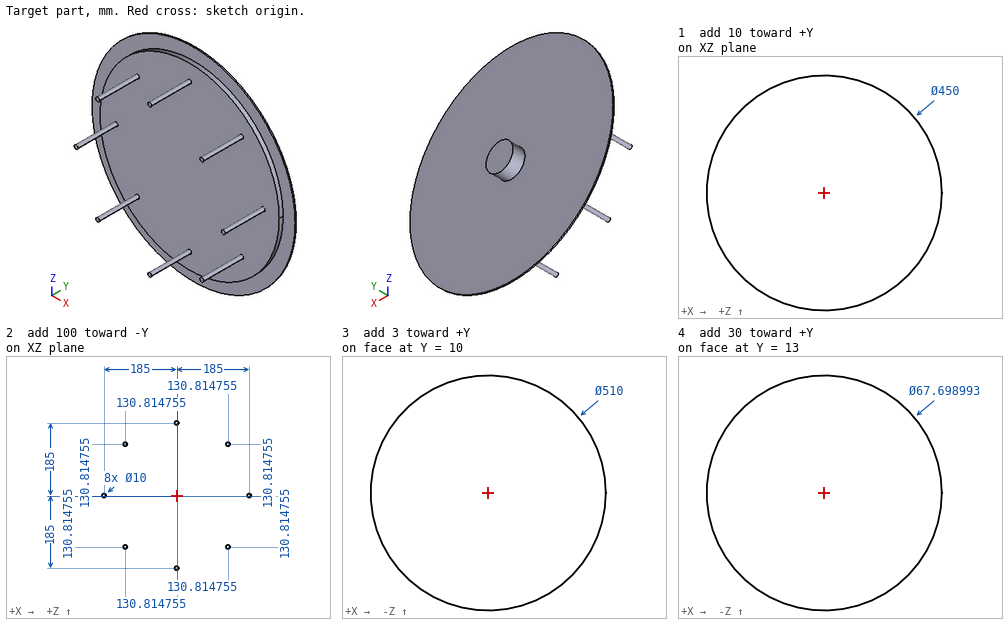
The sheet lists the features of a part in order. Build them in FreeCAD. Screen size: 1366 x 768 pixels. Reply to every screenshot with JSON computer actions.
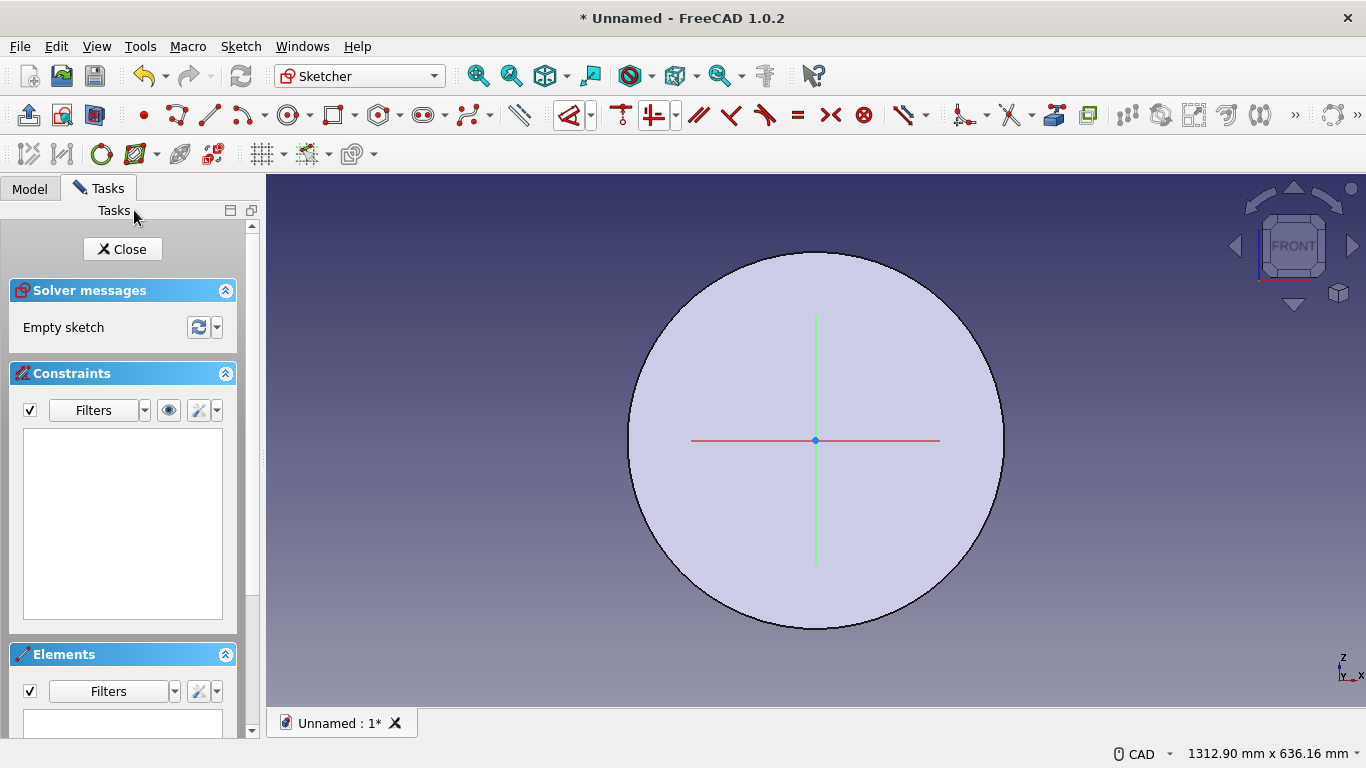
{"action": "left_click", "coordinate": [288, 116]}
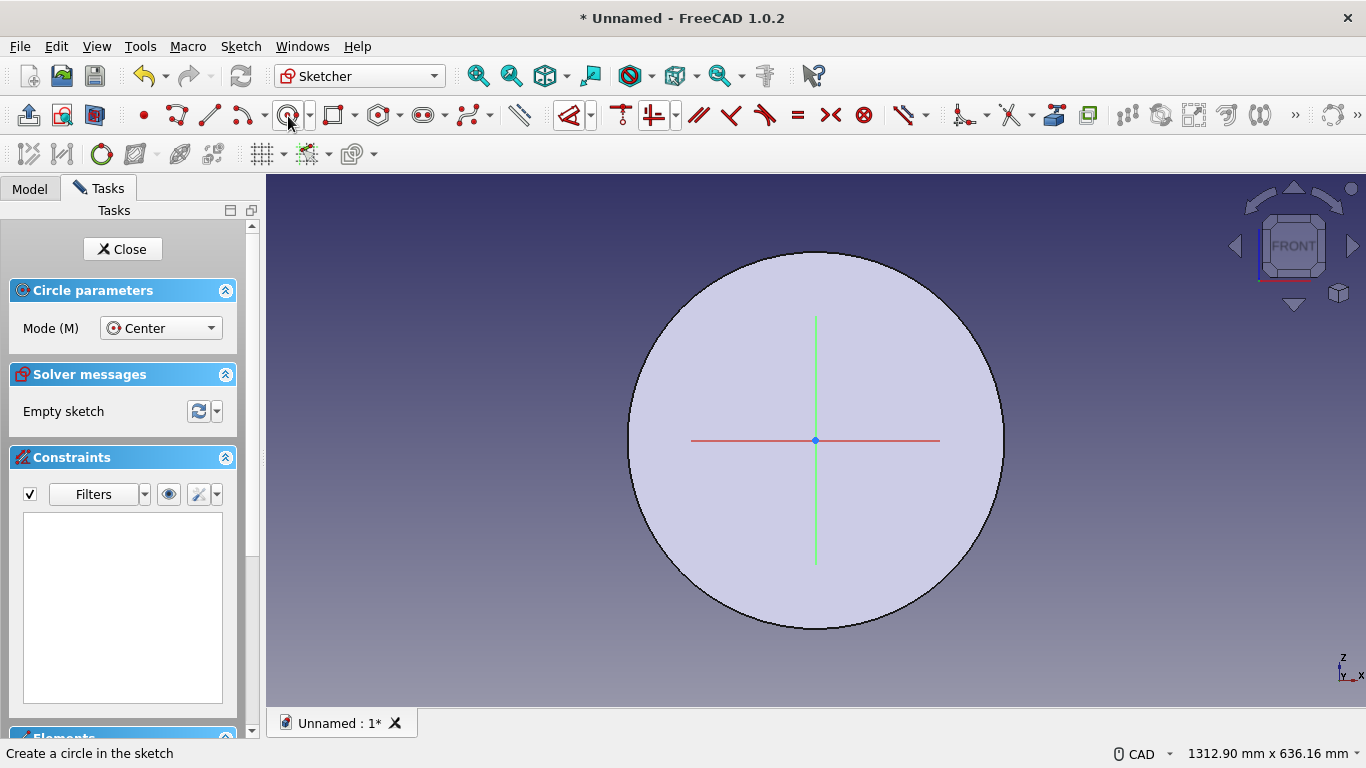
{"action": "scroll", "coordinate": [661, 440], "scroll_direction": "up", "scroll_amount": 9}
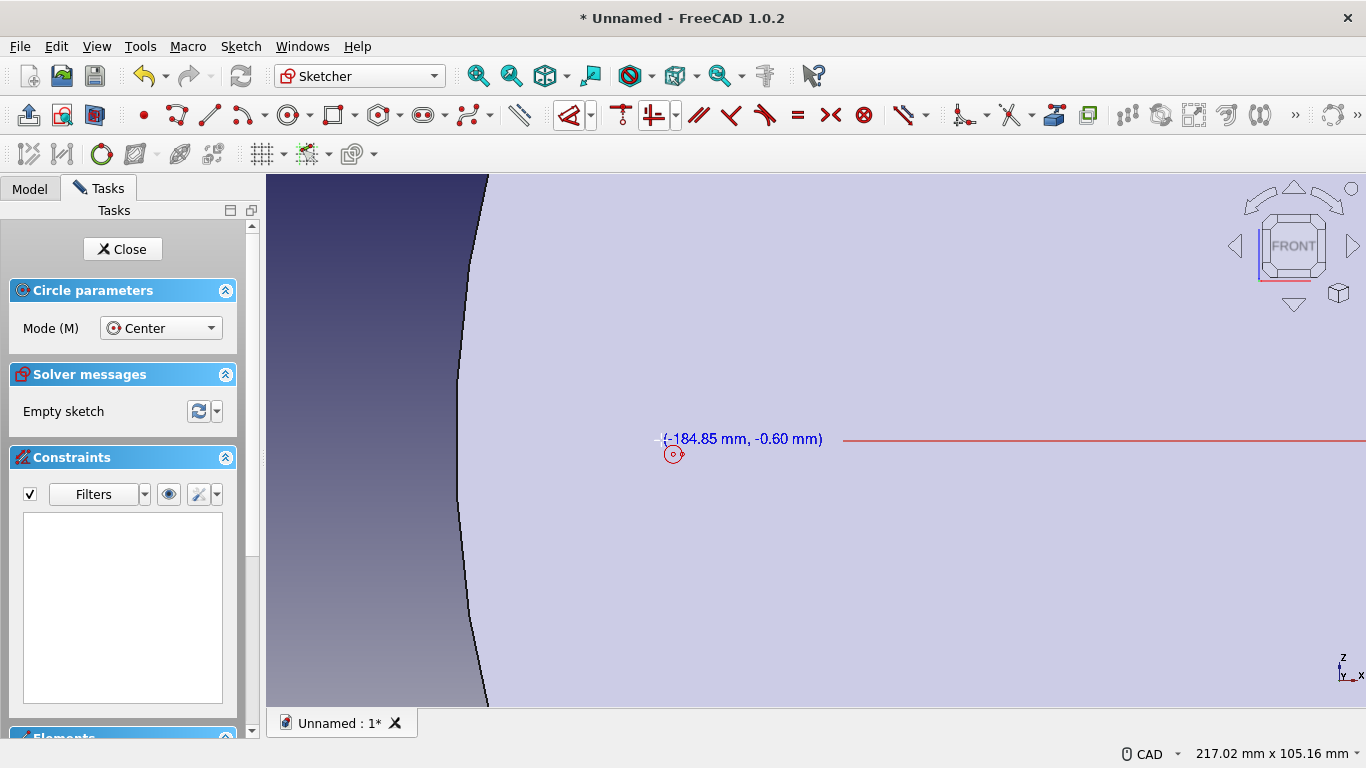
{"action": "scroll", "coordinate": [579, 440], "scroll_direction": "down", "scroll_amount": 9}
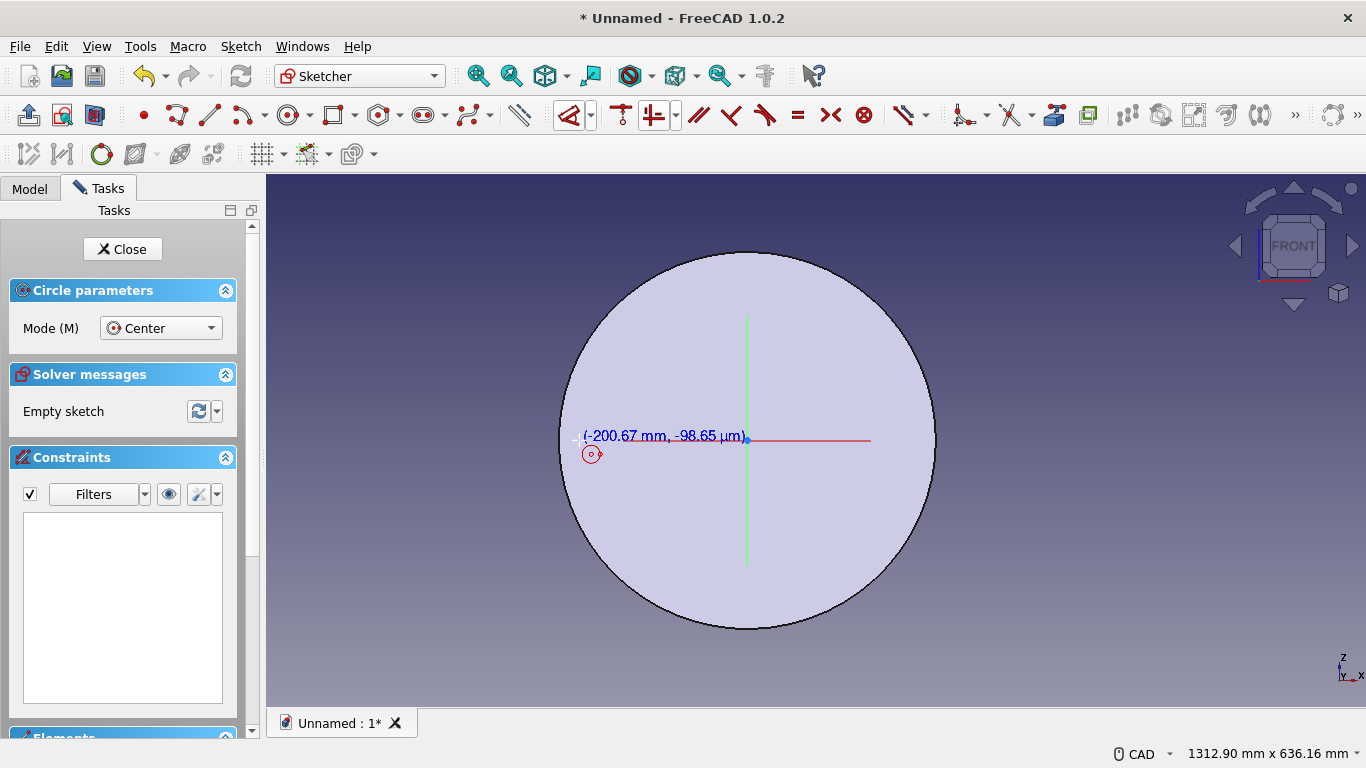
{"action": "left_click", "coordinate": [592, 440]}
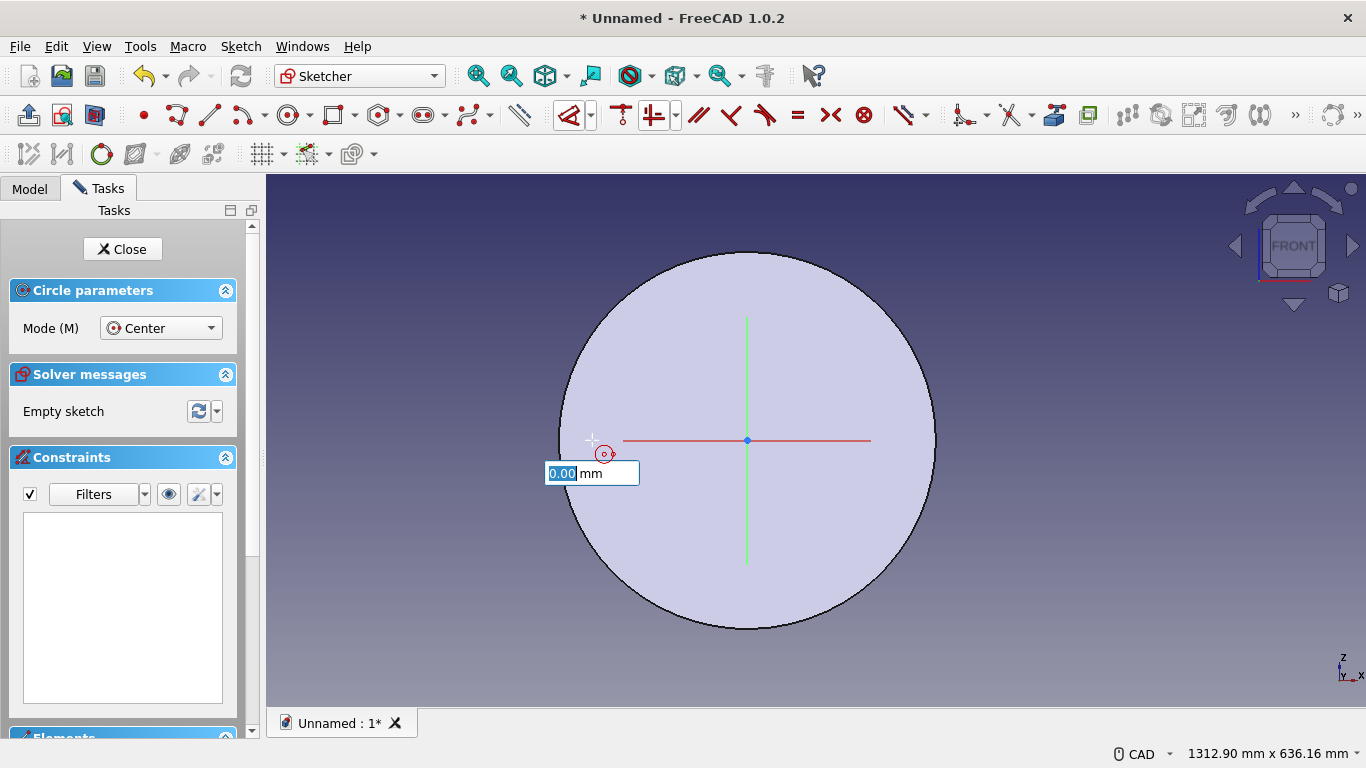
{"action": "scroll", "coordinate": [591, 444], "scroll_direction": "up", "scroll_amount": 7}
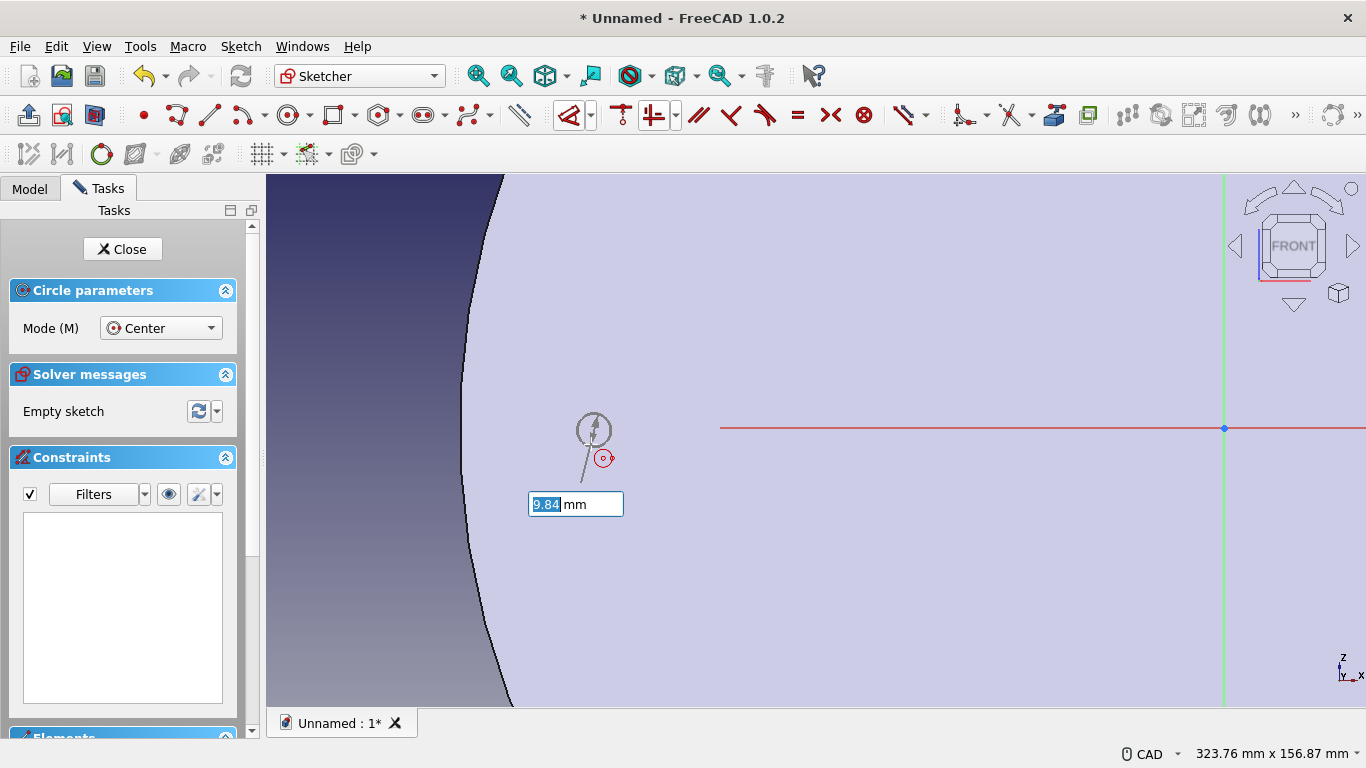
{"action": "left_click", "coordinate": [590, 444]}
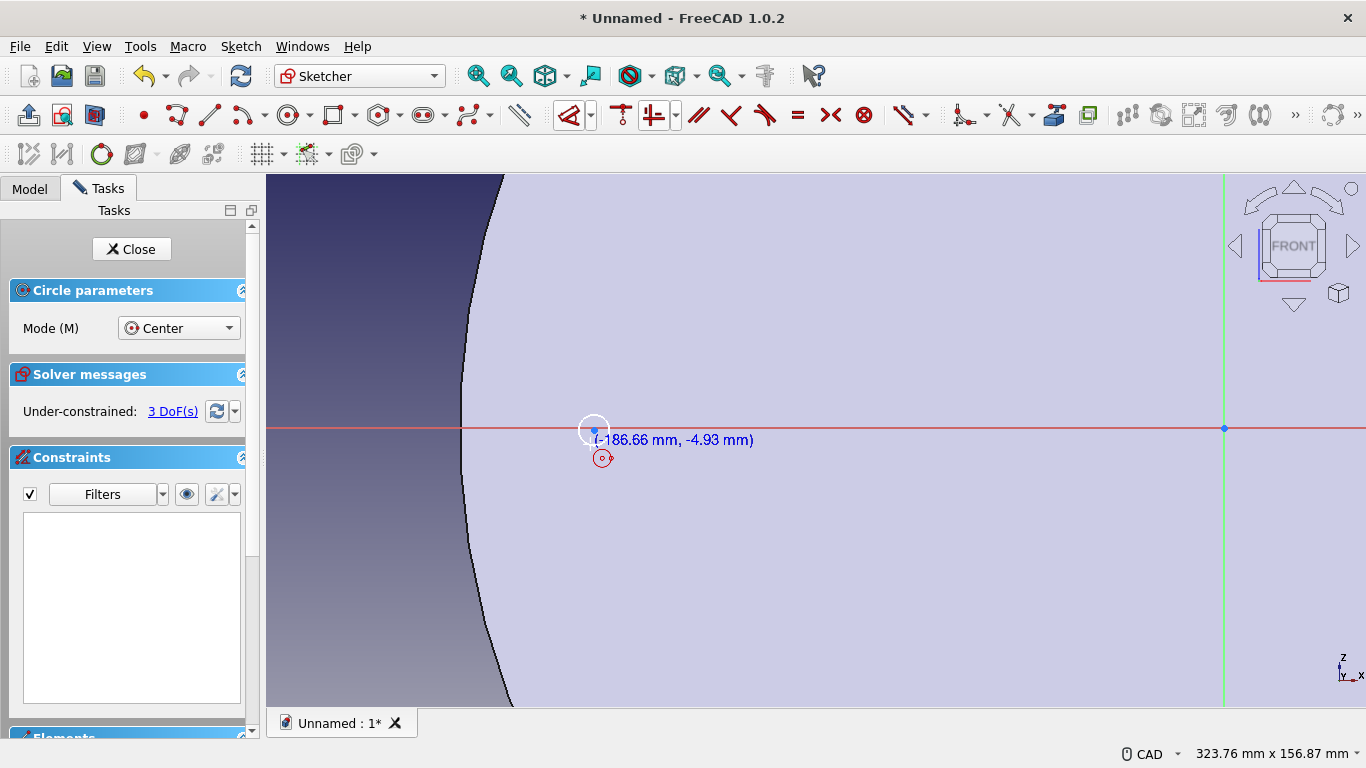
{"action": "scroll", "coordinate": [591, 445], "scroll_direction": "down", "scroll_amount": 7}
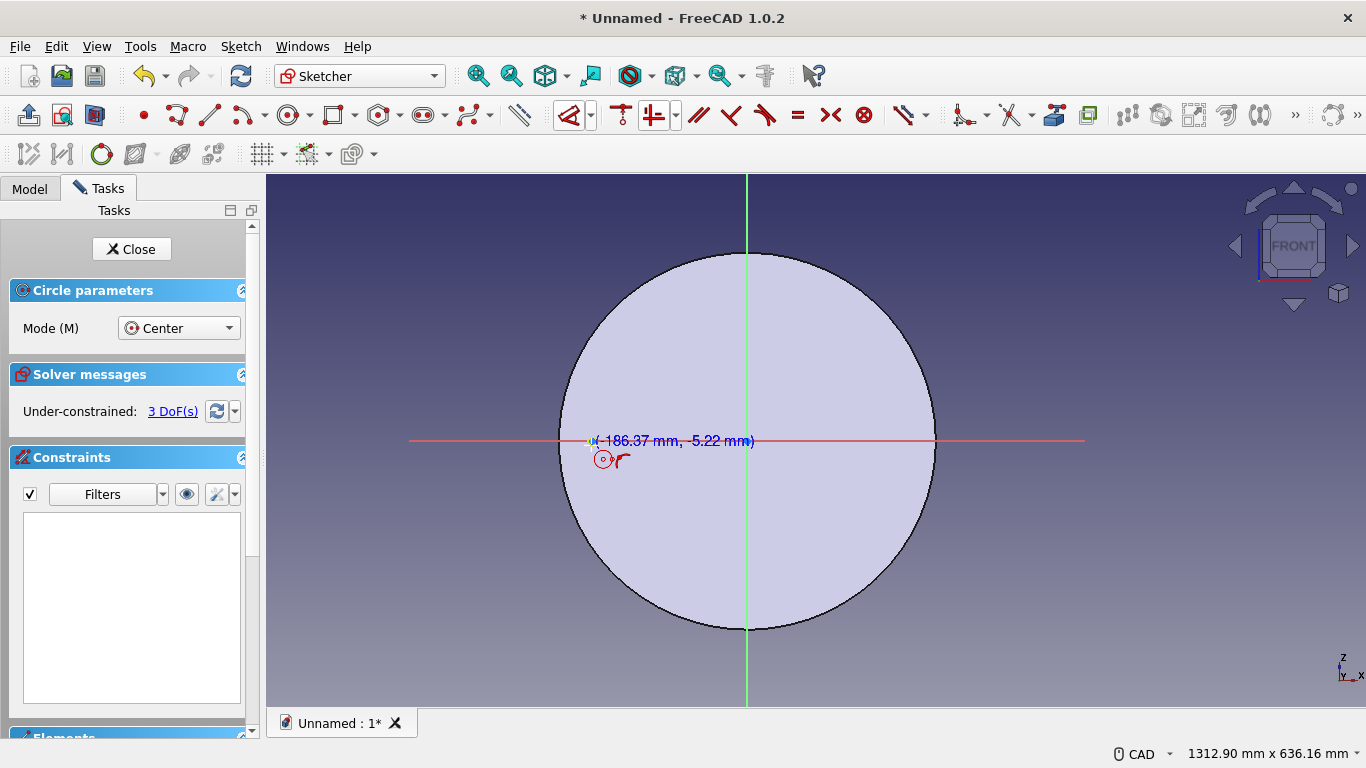
{"action": "scroll", "coordinate": [638, 332], "scroll_direction": "up", "scroll_amount": 9}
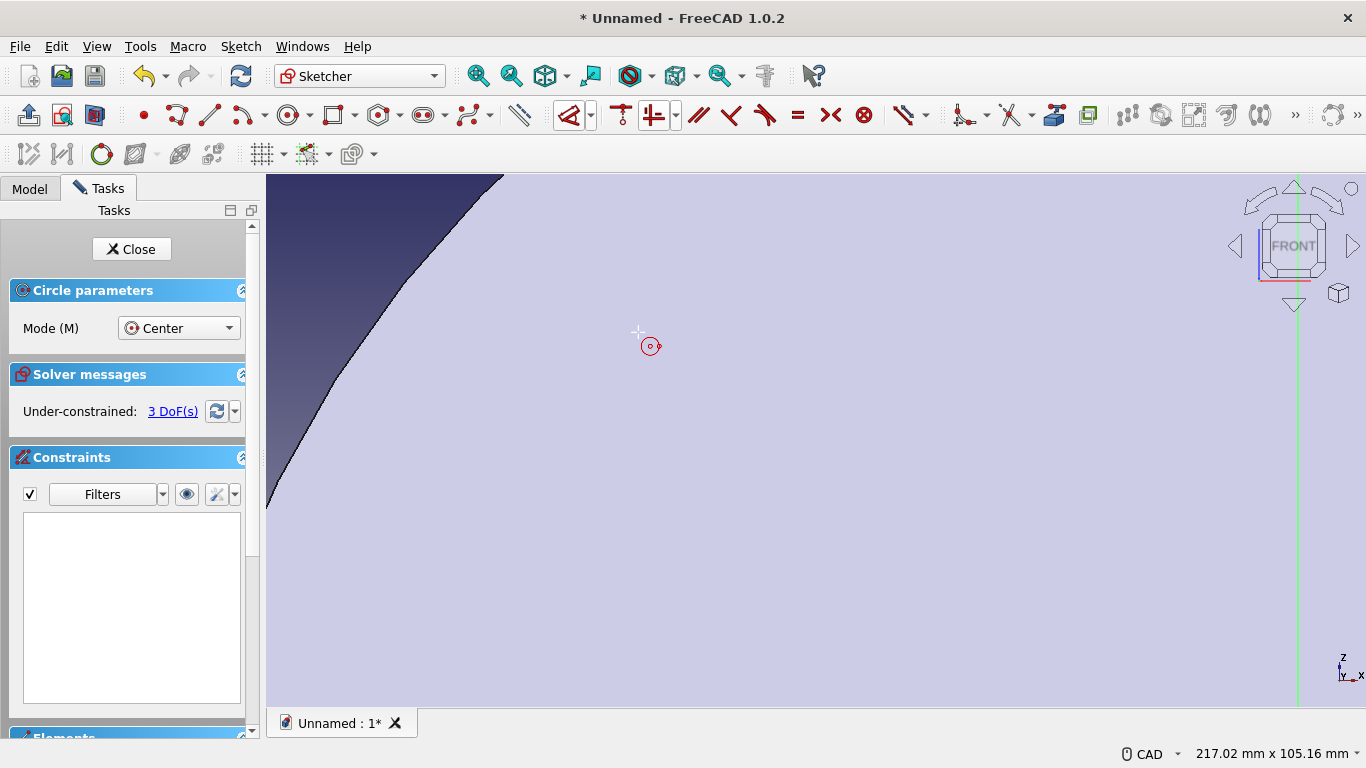
{"action": "scroll", "coordinate": [638, 331], "scroll_direction": "down", "scroll_amount": 9}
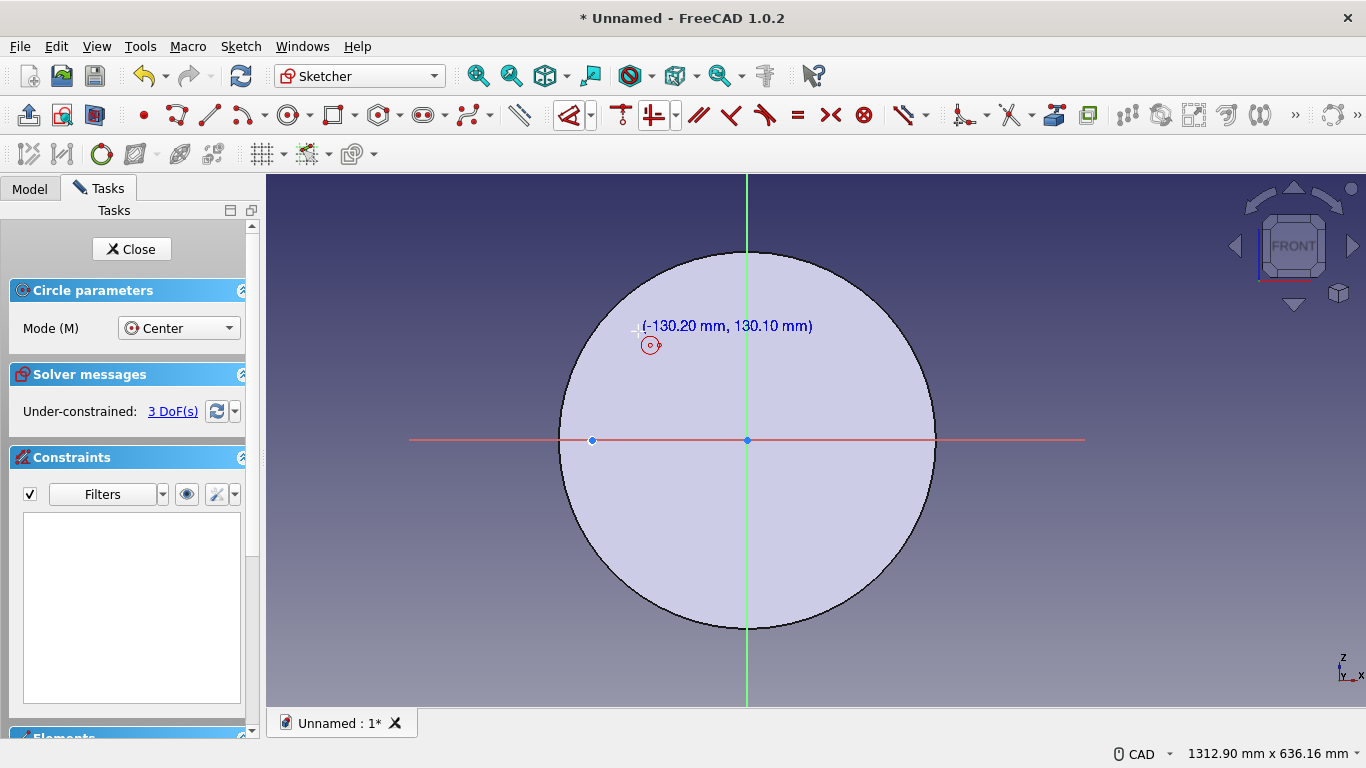
{"action": "left_click", "coordinate": [638, 331]}